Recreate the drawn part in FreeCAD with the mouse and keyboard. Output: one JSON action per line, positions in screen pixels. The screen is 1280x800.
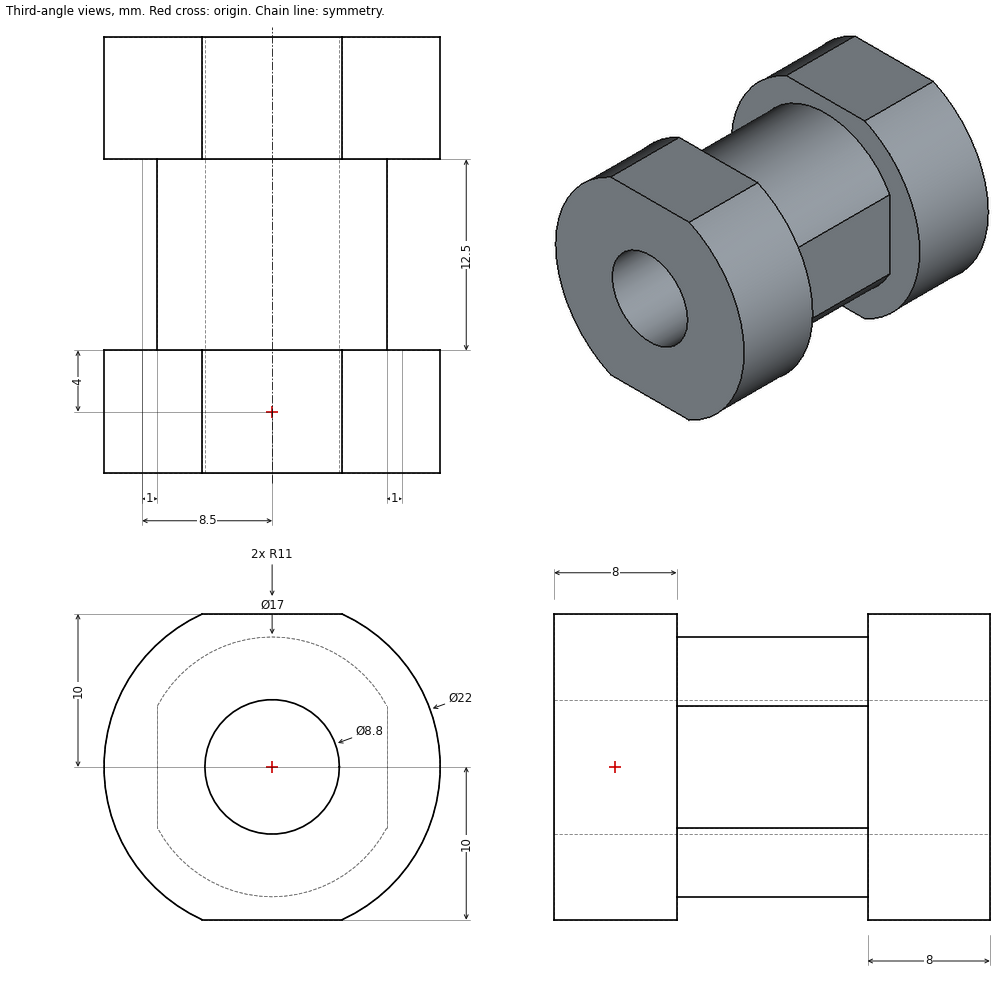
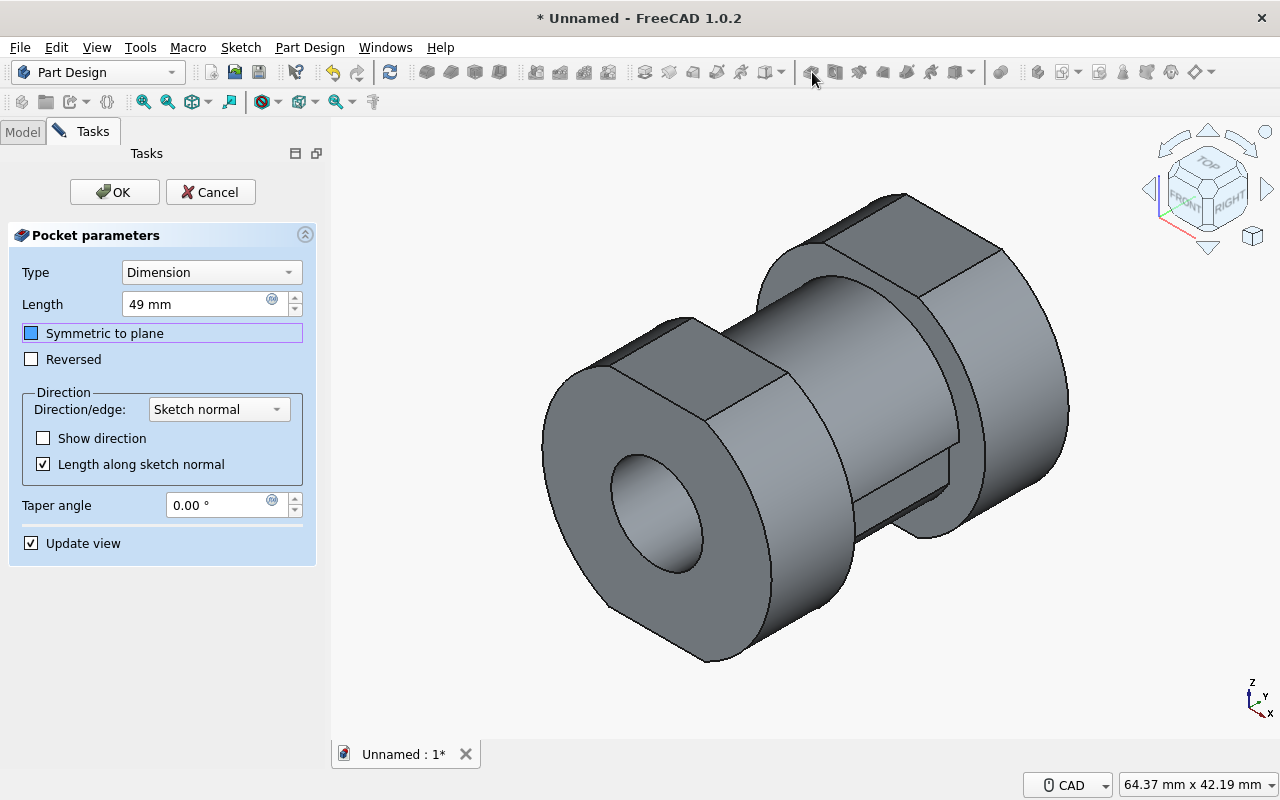
{"action": "left_click", "coordinate": [30, 333]}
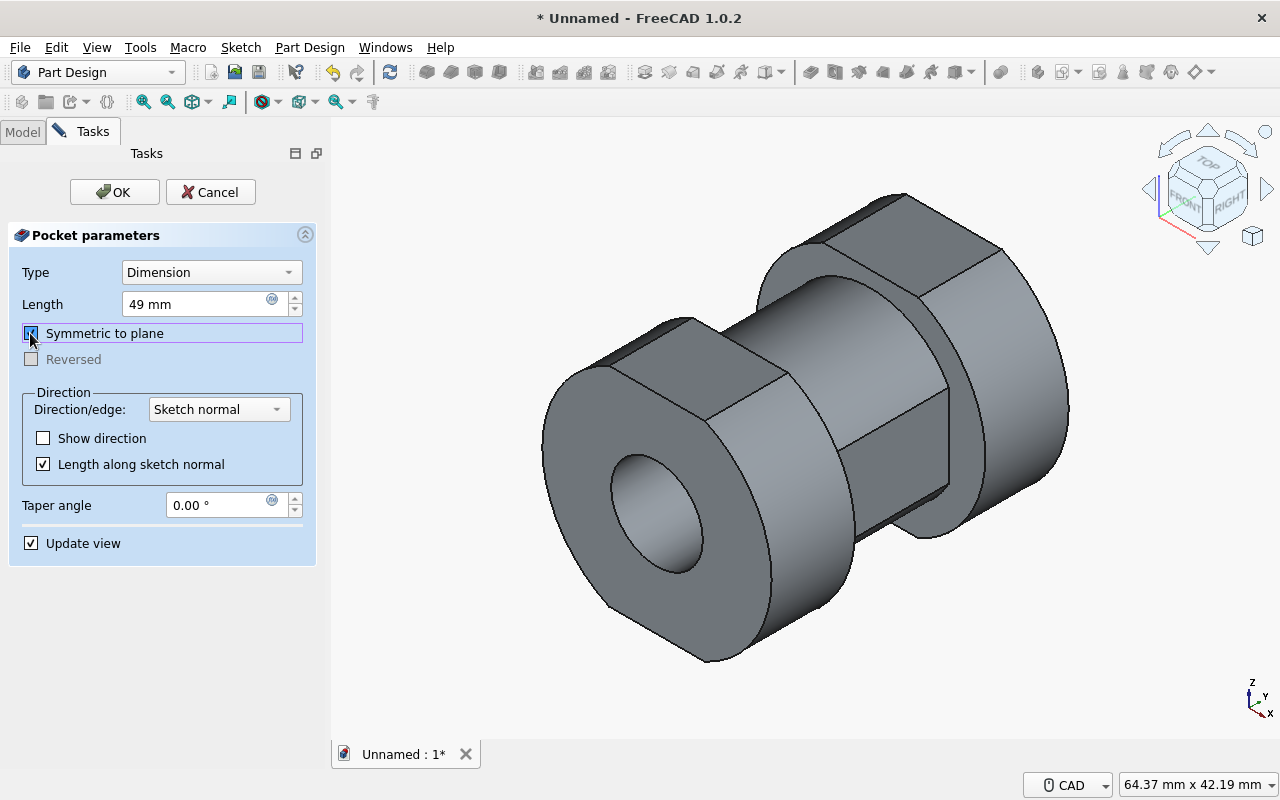
{"action": "left_click", "coordinate": [115, 192]}